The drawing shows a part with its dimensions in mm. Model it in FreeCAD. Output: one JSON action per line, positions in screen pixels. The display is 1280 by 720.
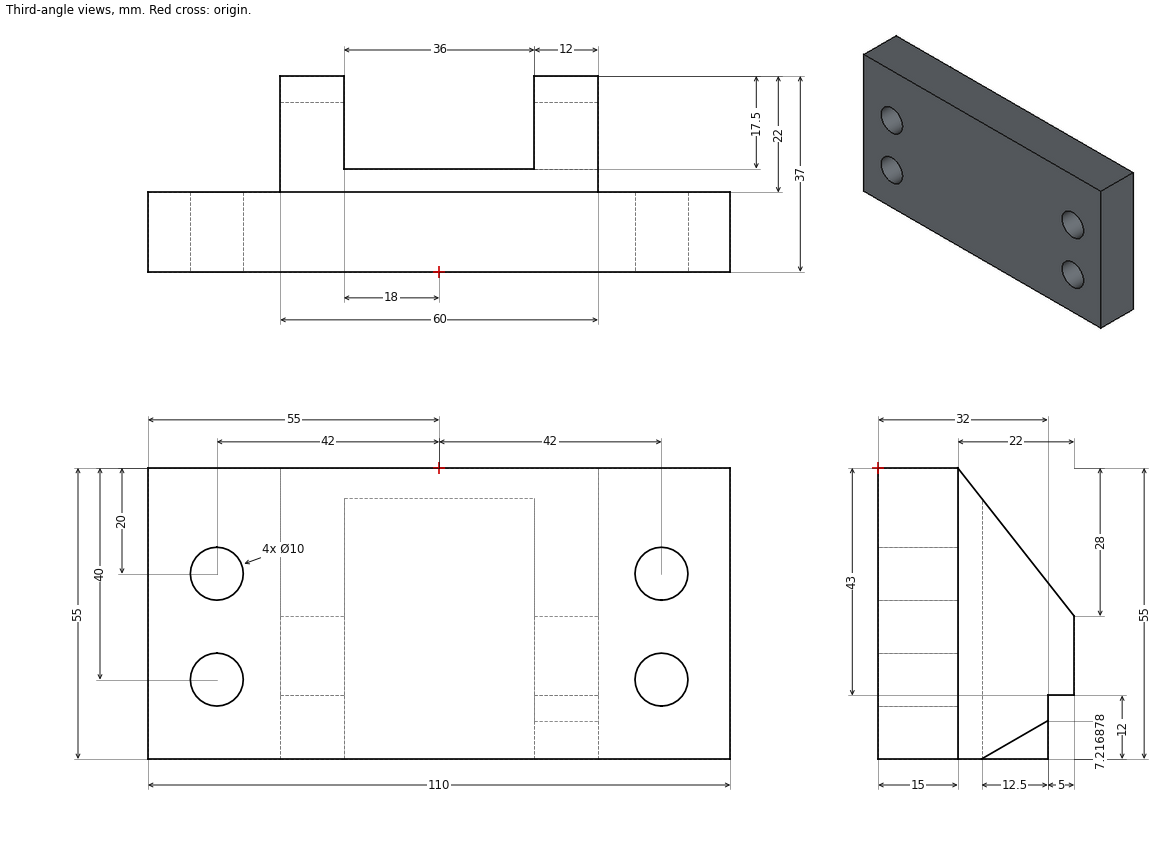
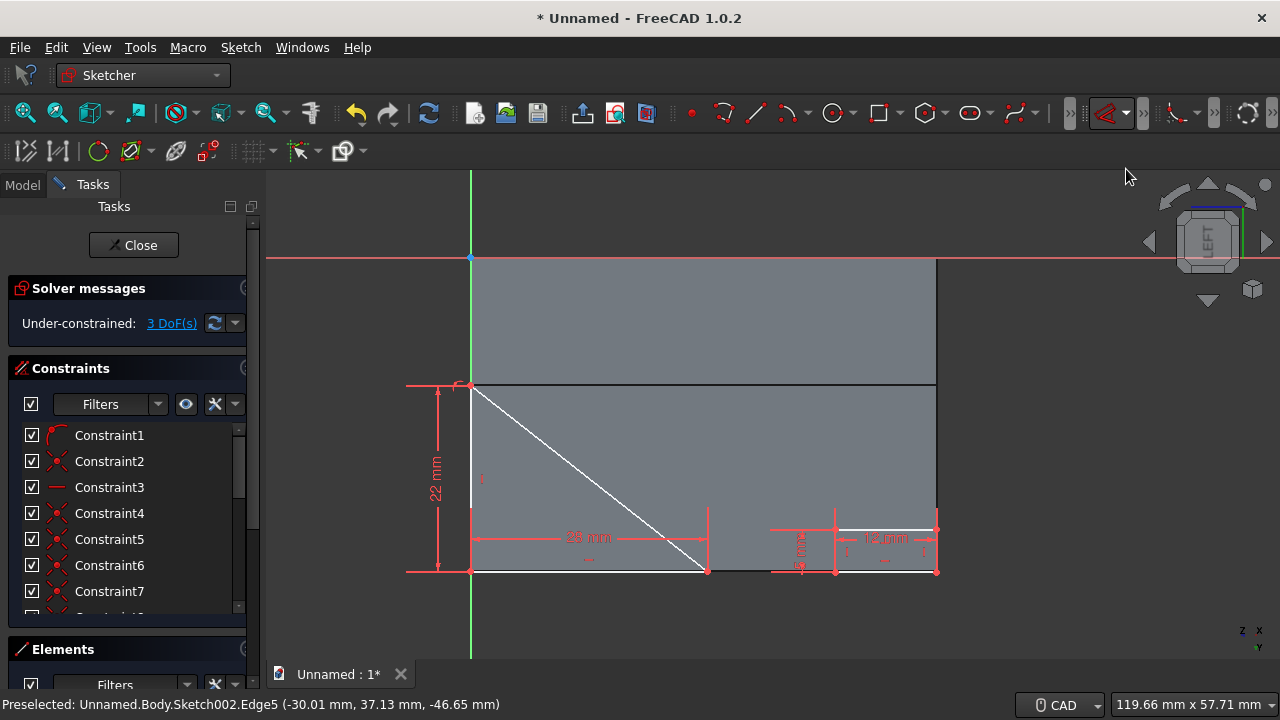
{"action": "left_click", "coordinate": [471, 386]}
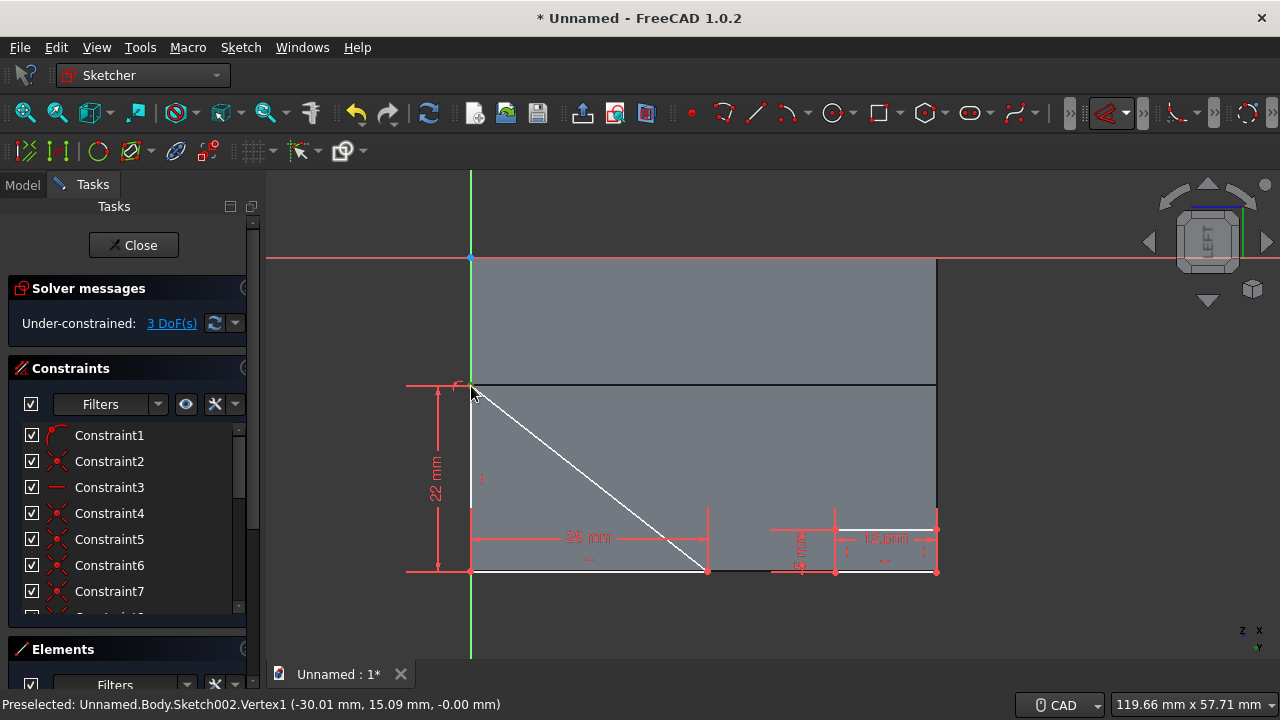
{"action": "key", "text": "i"}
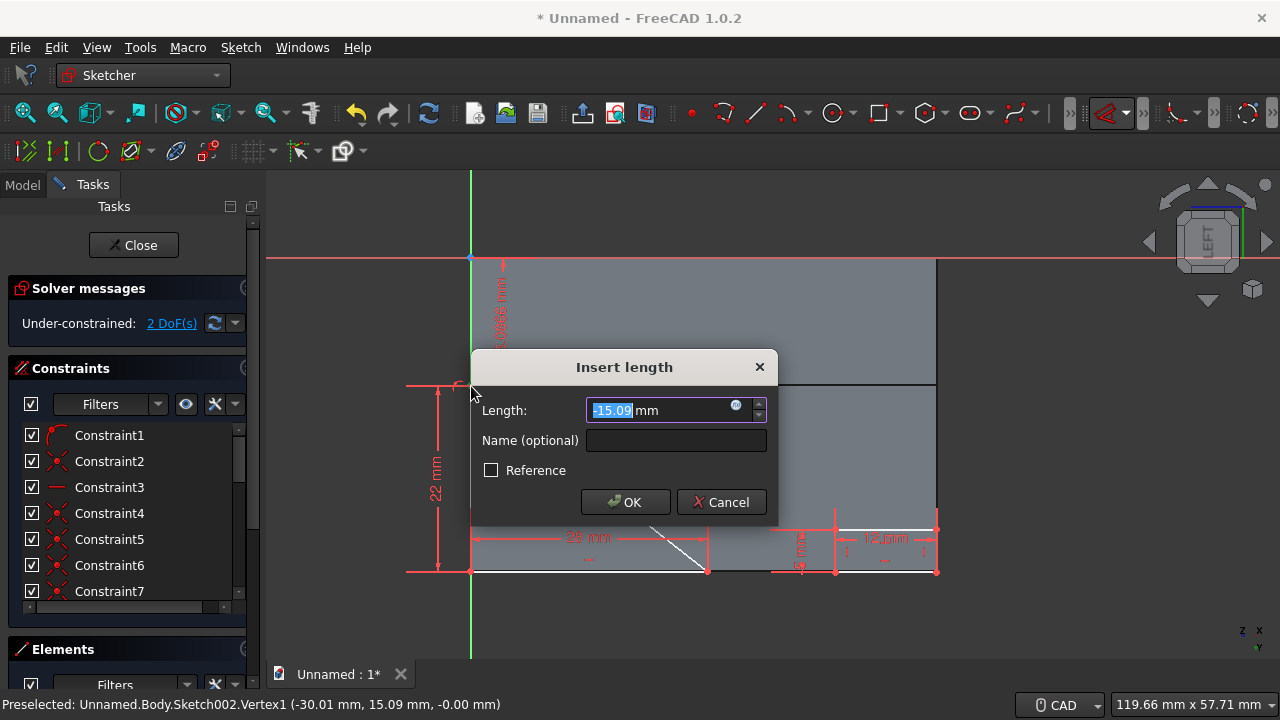
{"action": "type", "text": "-15"}
{"action": "key", "text": "Return"}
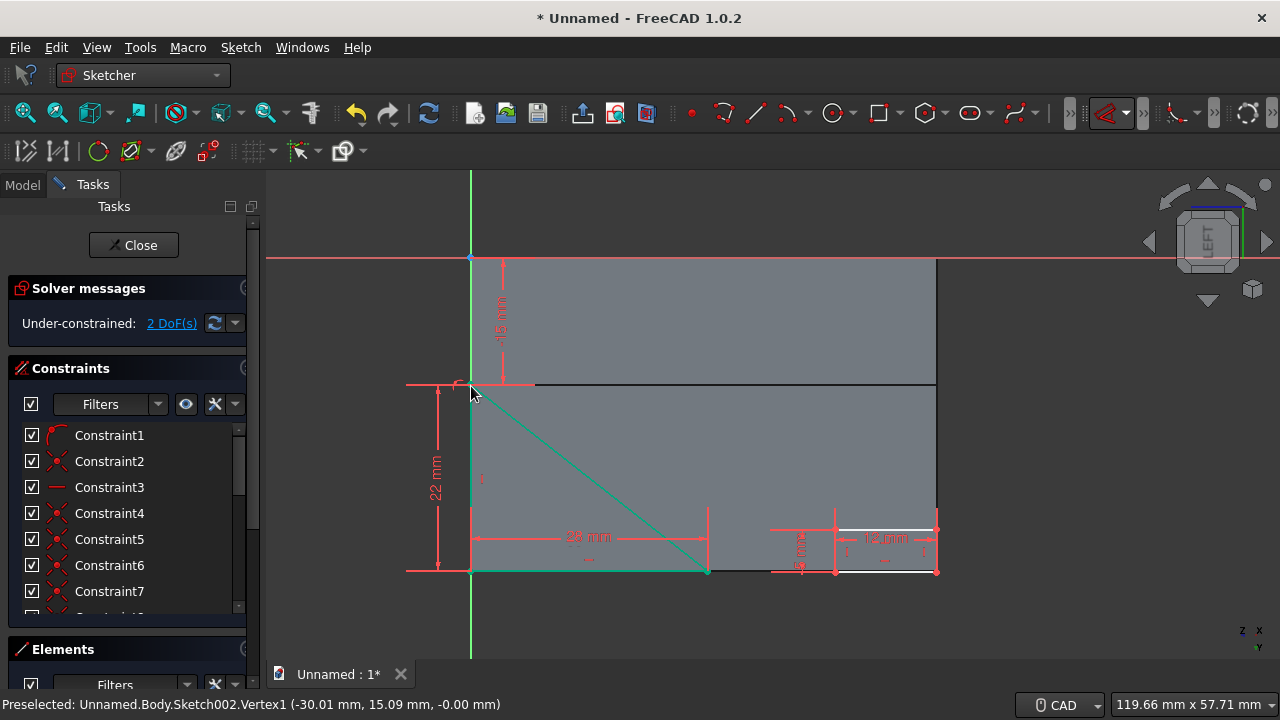
{"action": "left_click", "coordinate": [835, 530]}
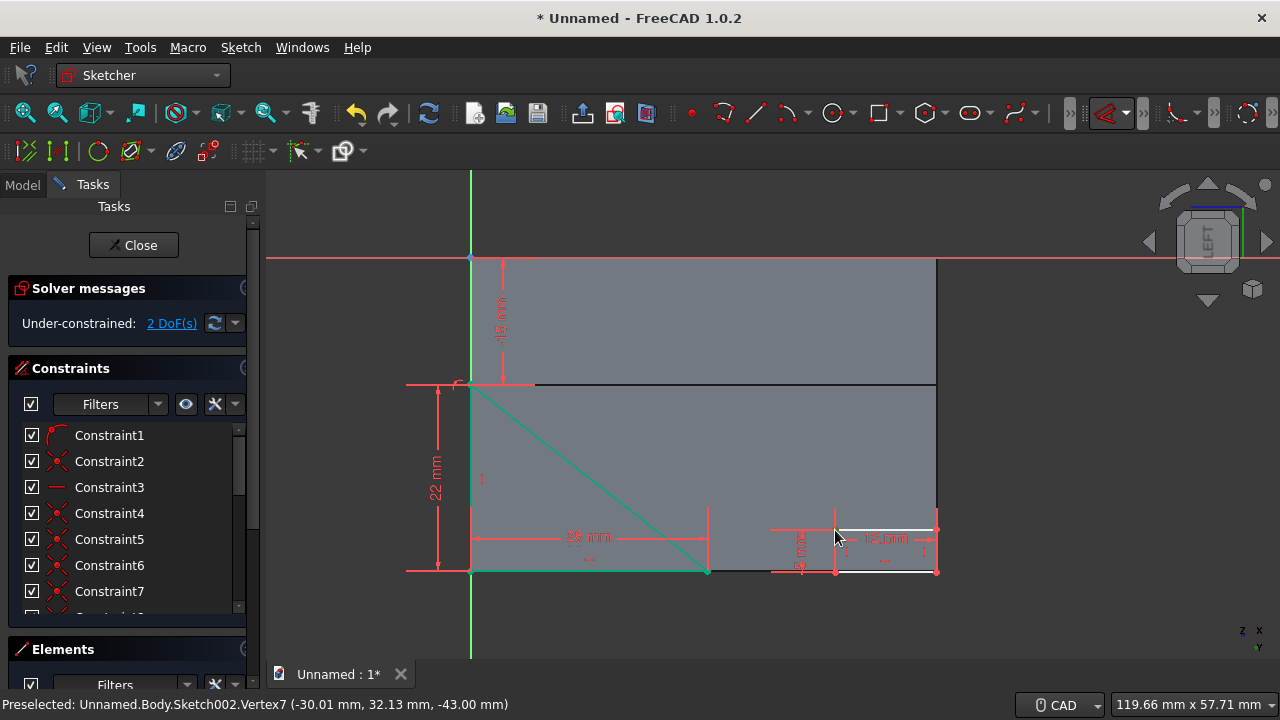
{"action": "key", "text": "l"}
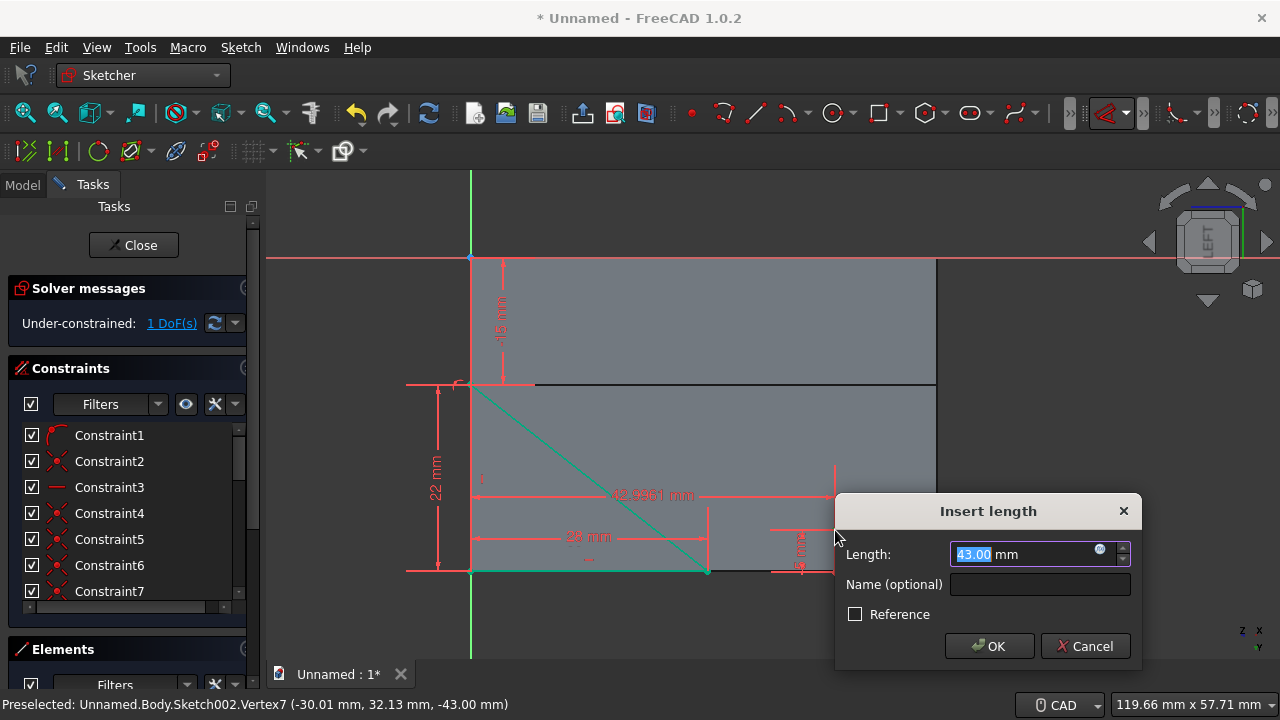
{"action": "type", "text": "43"}
{"action": "key", "text": "Return"}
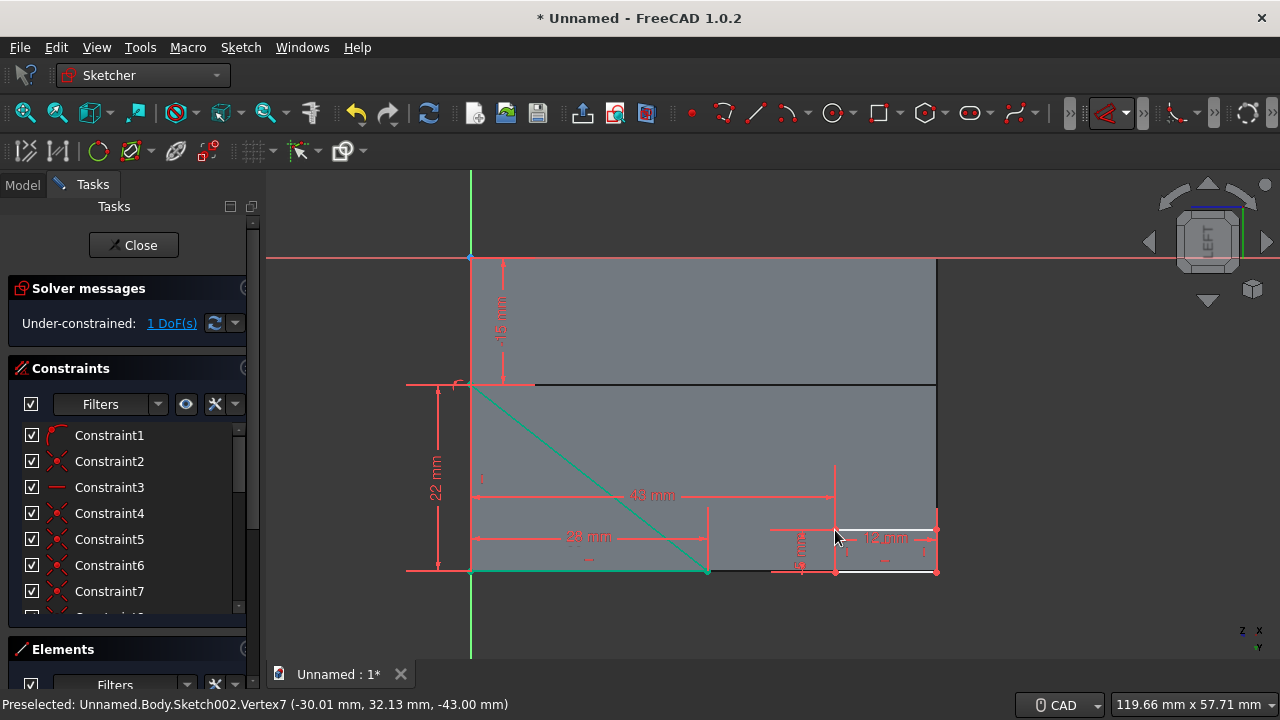
{"action": "left_click", "coordinate": [835, 530]}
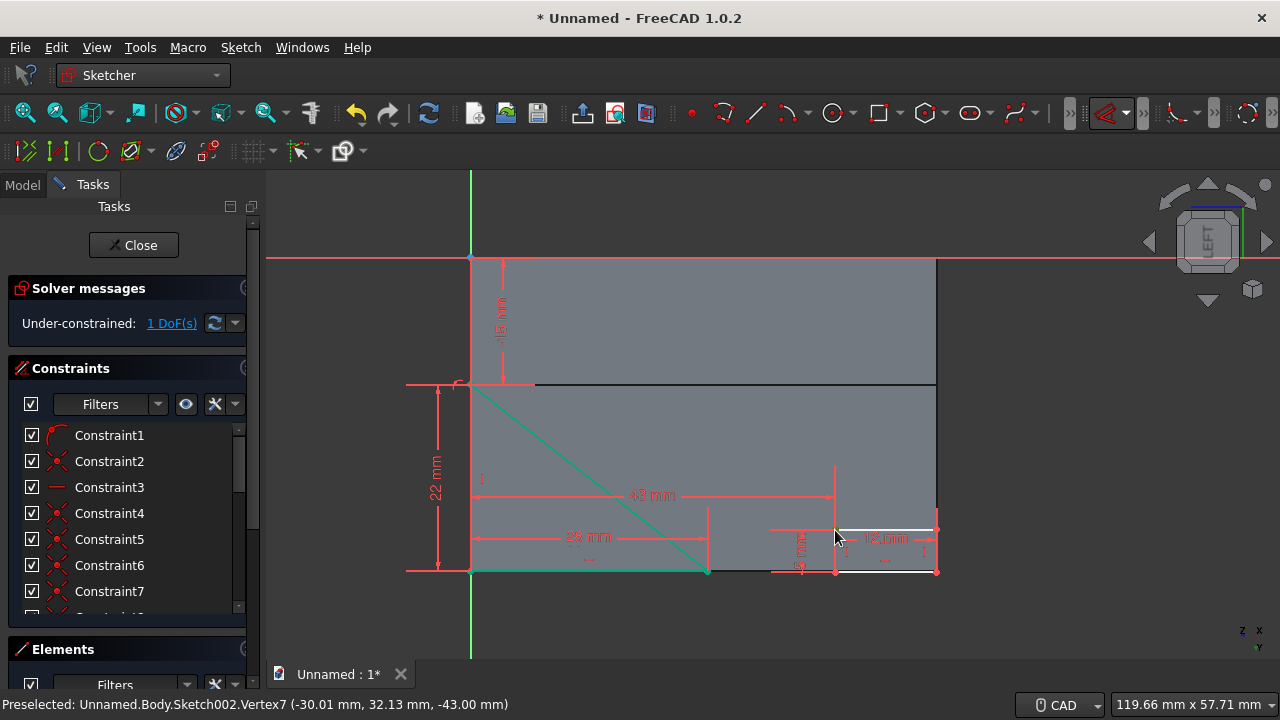
{"action": "left_click", "coordinate": [1128, 114]}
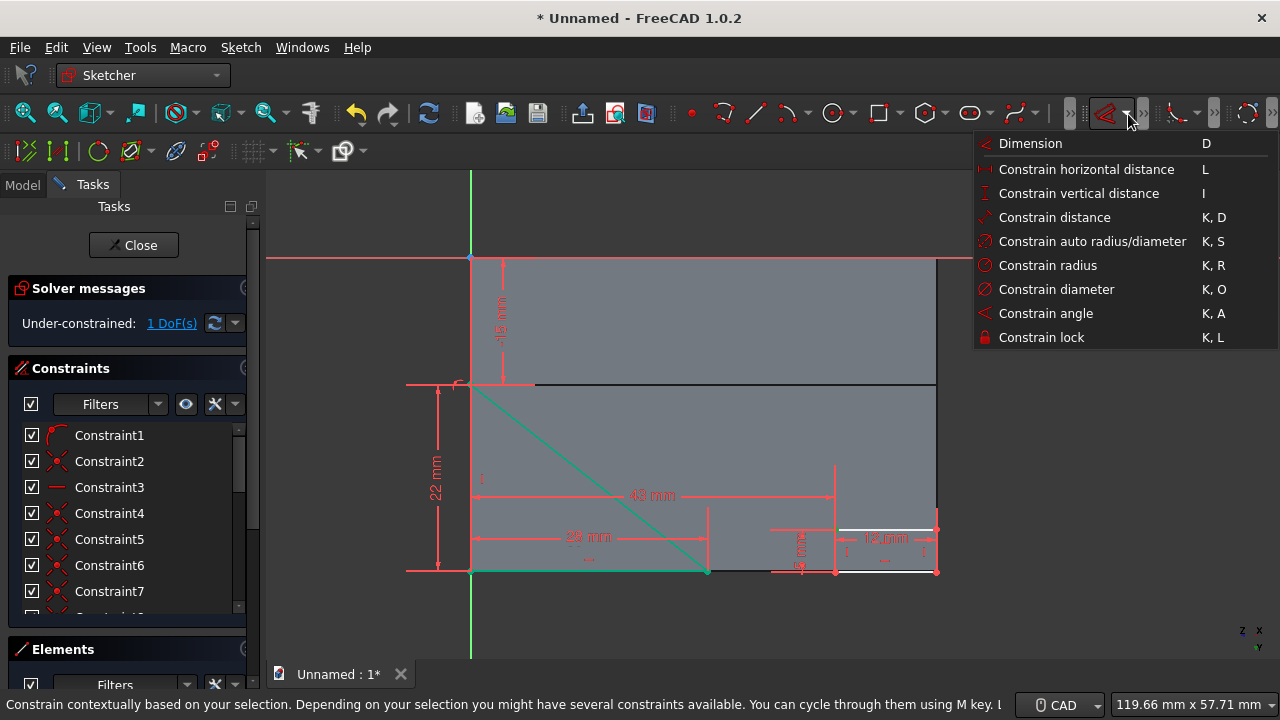
{"action": "left_click", "coordinate": [1126, 193]}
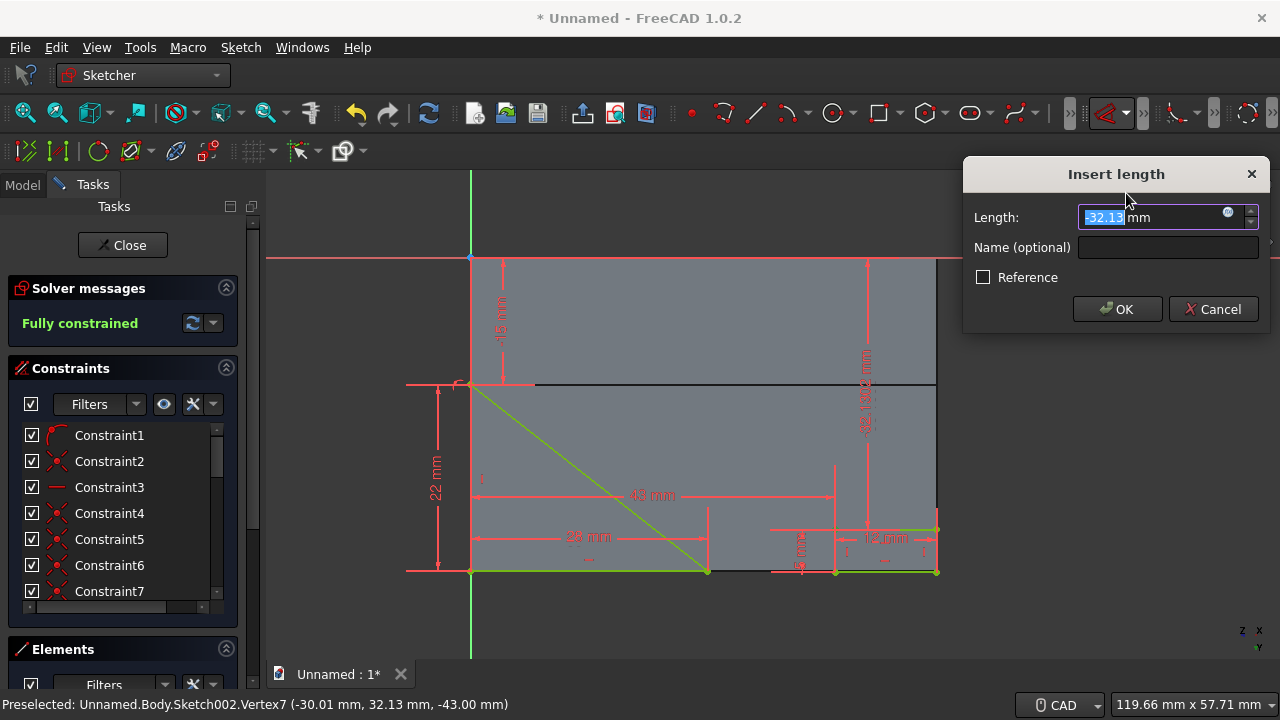
{"action": "type", "text": "-32"}
{"action": "key", "text": "Return"}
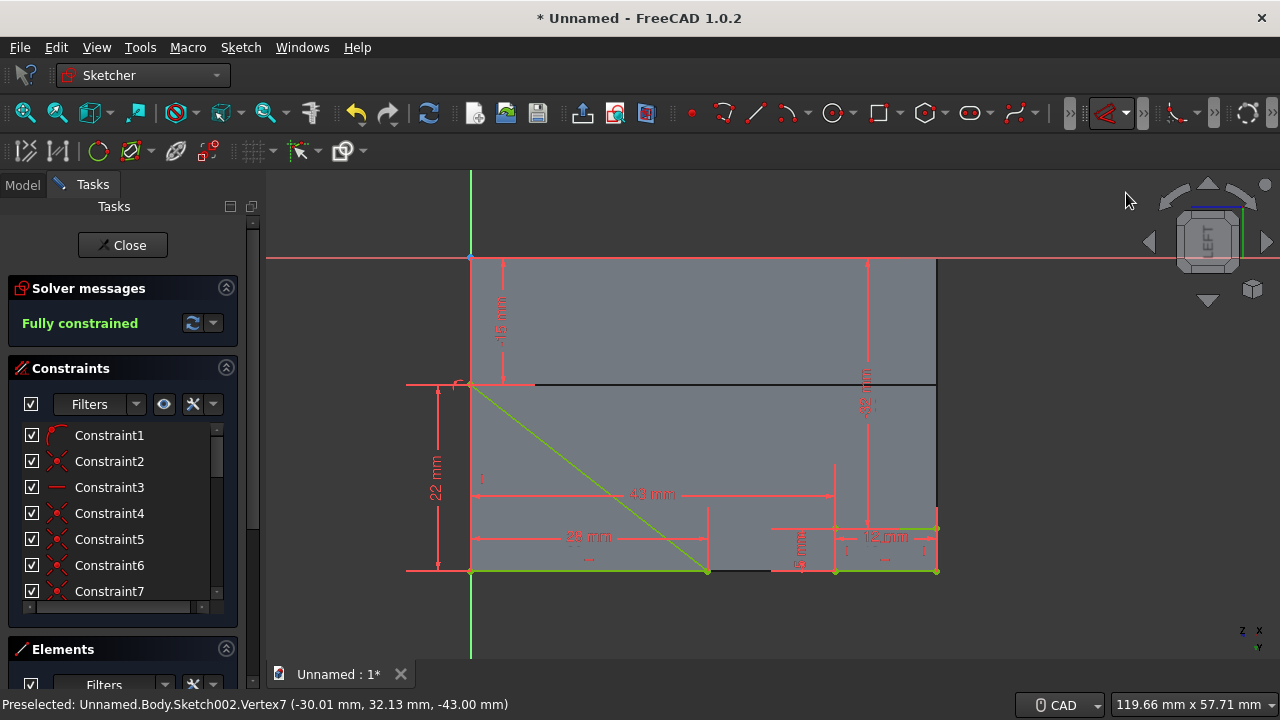
{"action": "left_click", "coordinate": [123, 245]}